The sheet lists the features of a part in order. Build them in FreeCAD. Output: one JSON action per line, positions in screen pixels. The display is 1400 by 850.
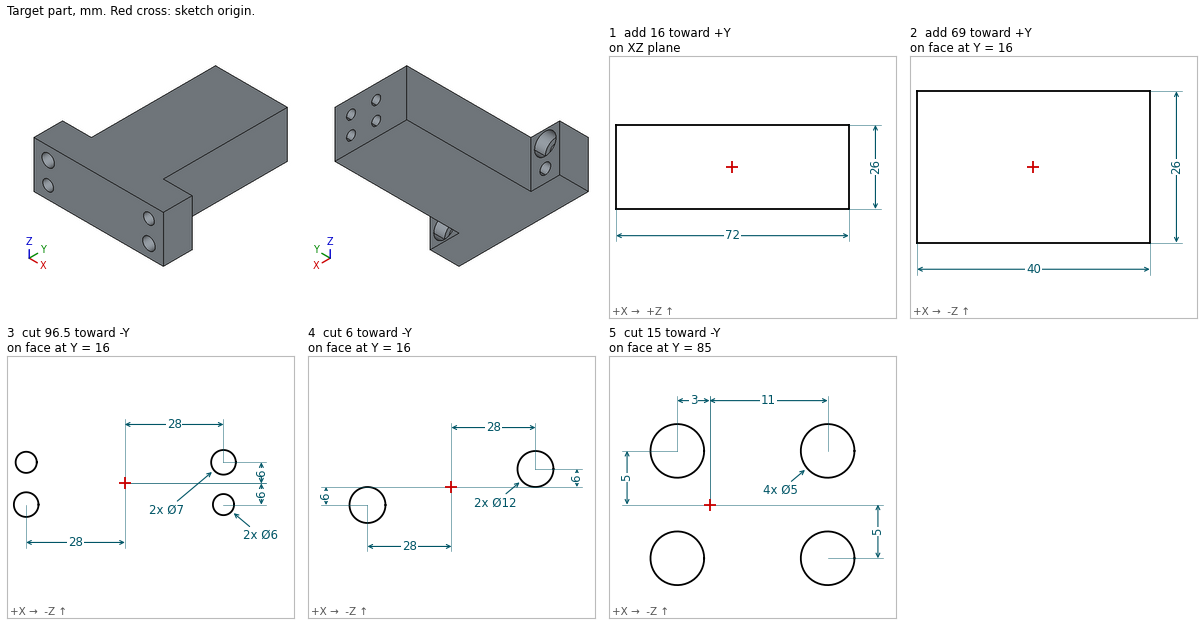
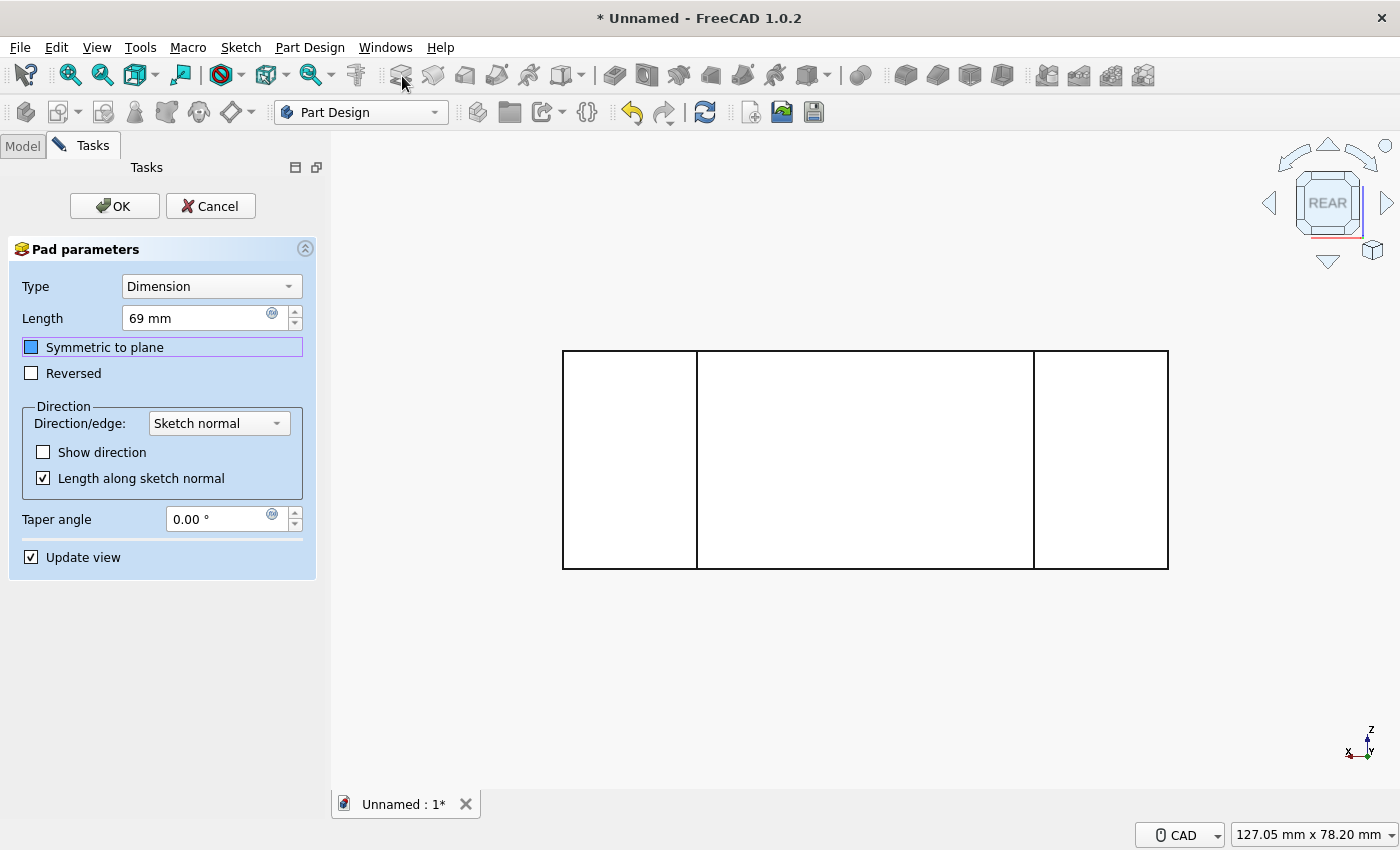
{"action": "left_click", "coordinate": [115, 206]}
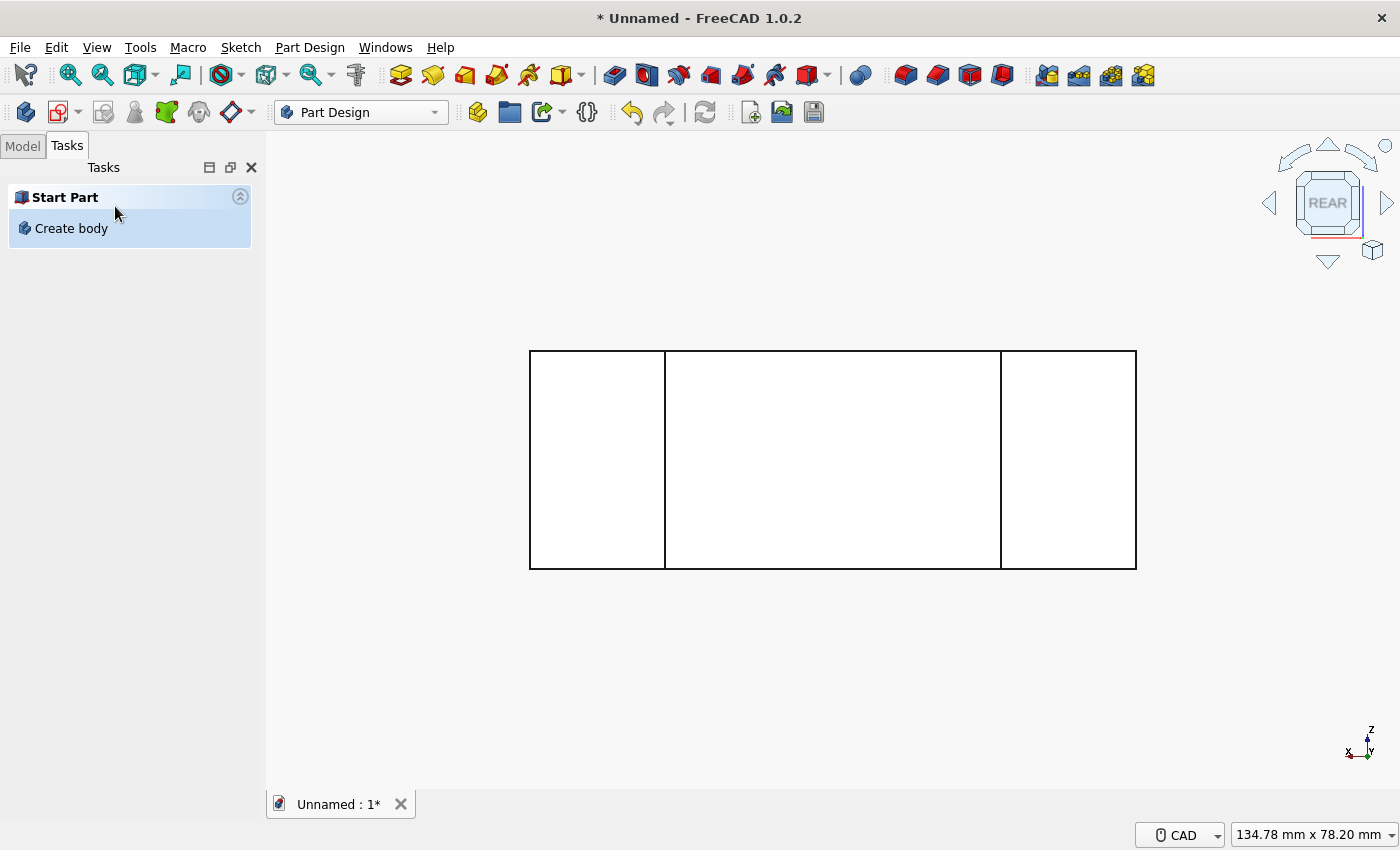
{"action": "left_click", "coordinate": [597, 428]}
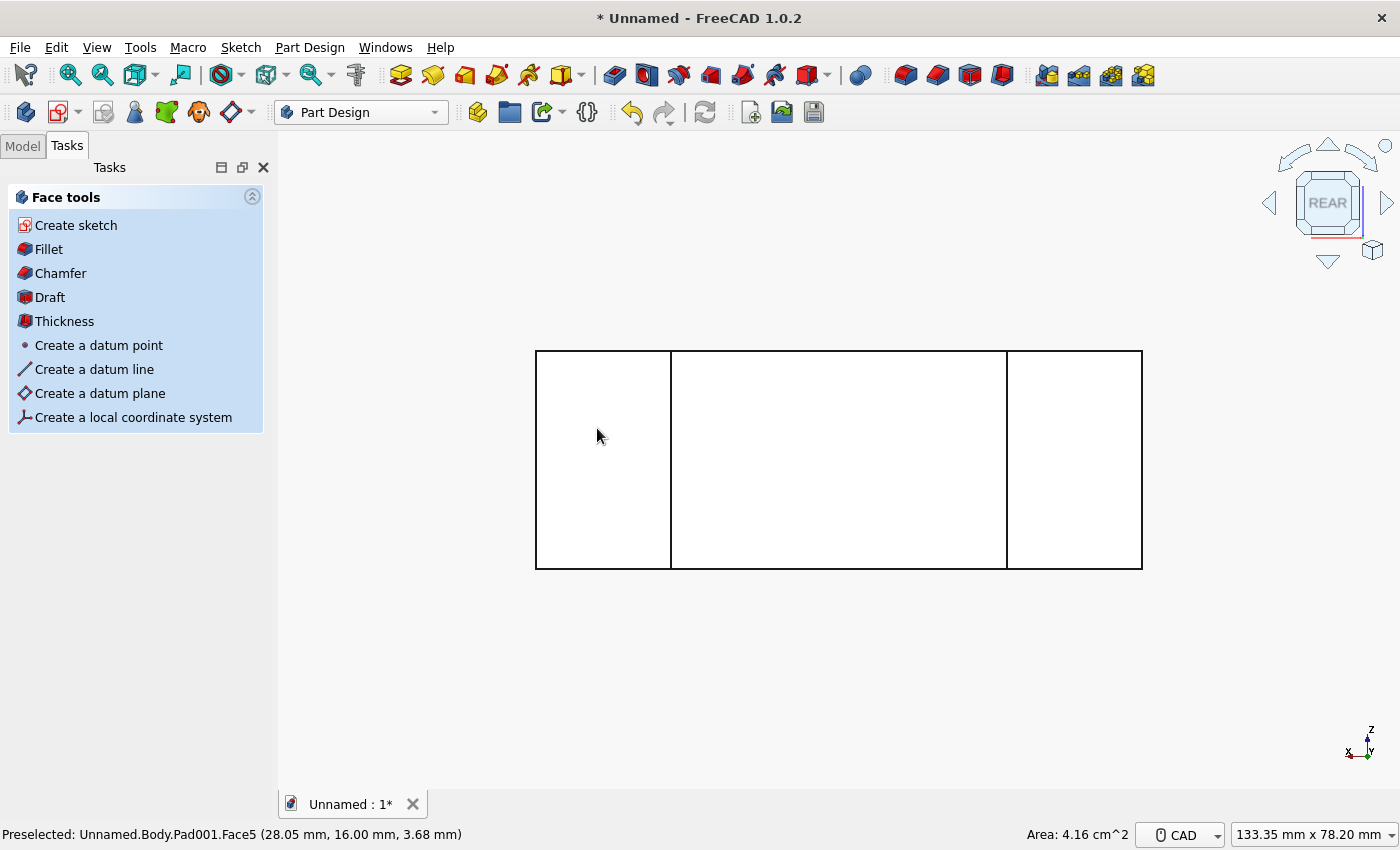
{"action": "left_click", "coordinate": [58, 112]}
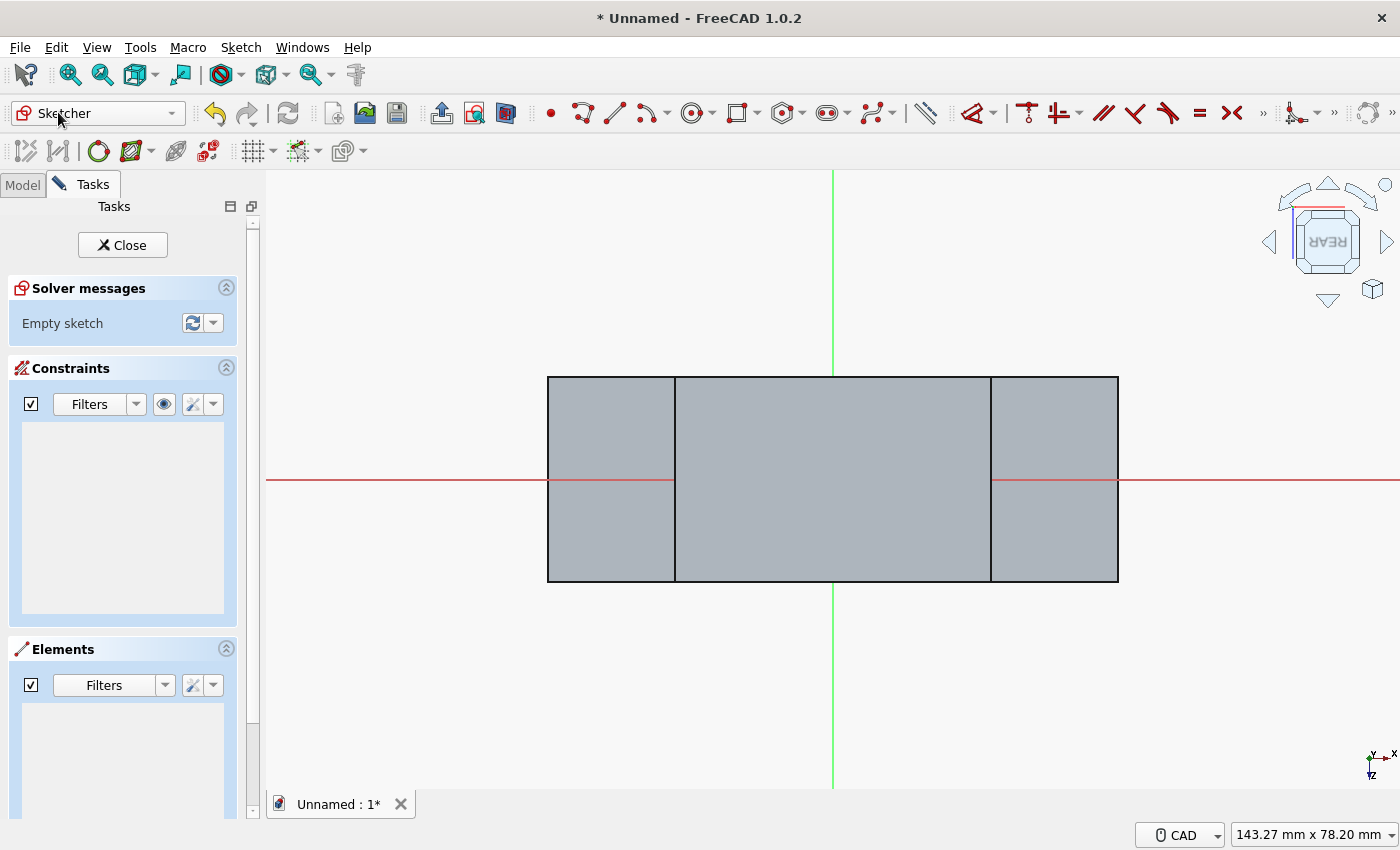
{"action": "key", "text": "g c"}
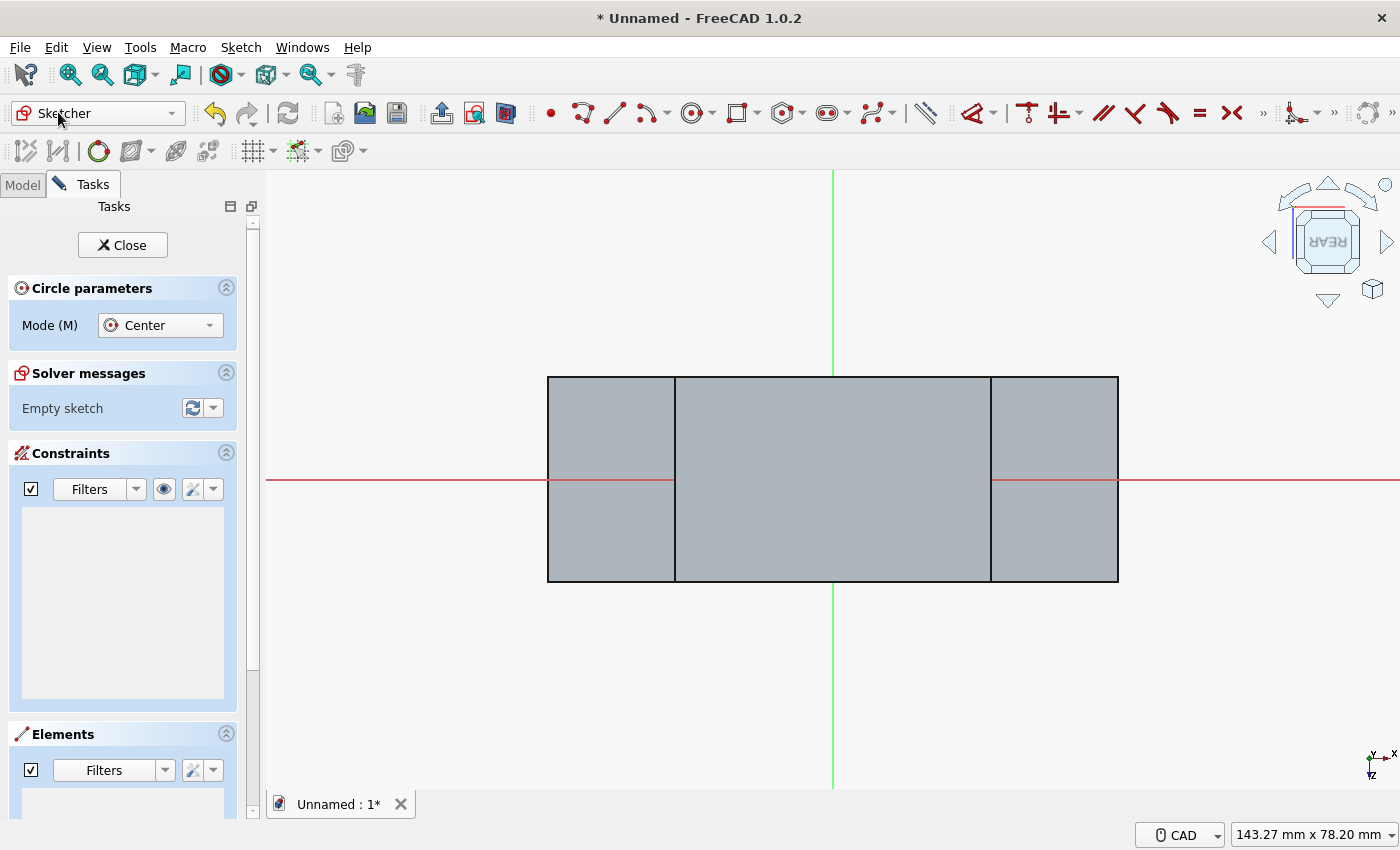
{"action": "left_click", "coordinate": [1055, 432]}
{"action": "mouse_move", "coordinate": [1074, 412]}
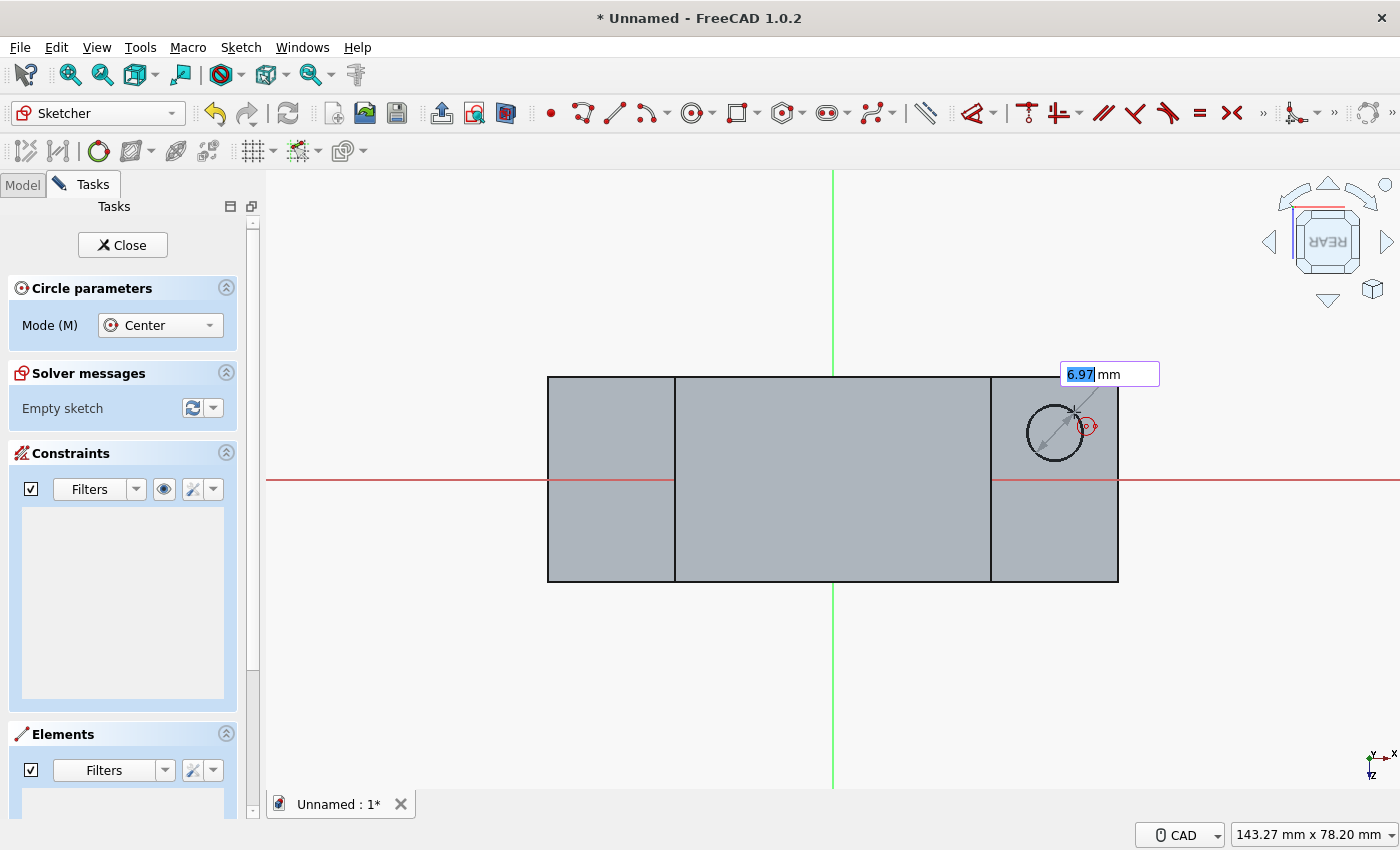
{"action": "type", "text": "7"}
{"action": "key", "text": "Return"}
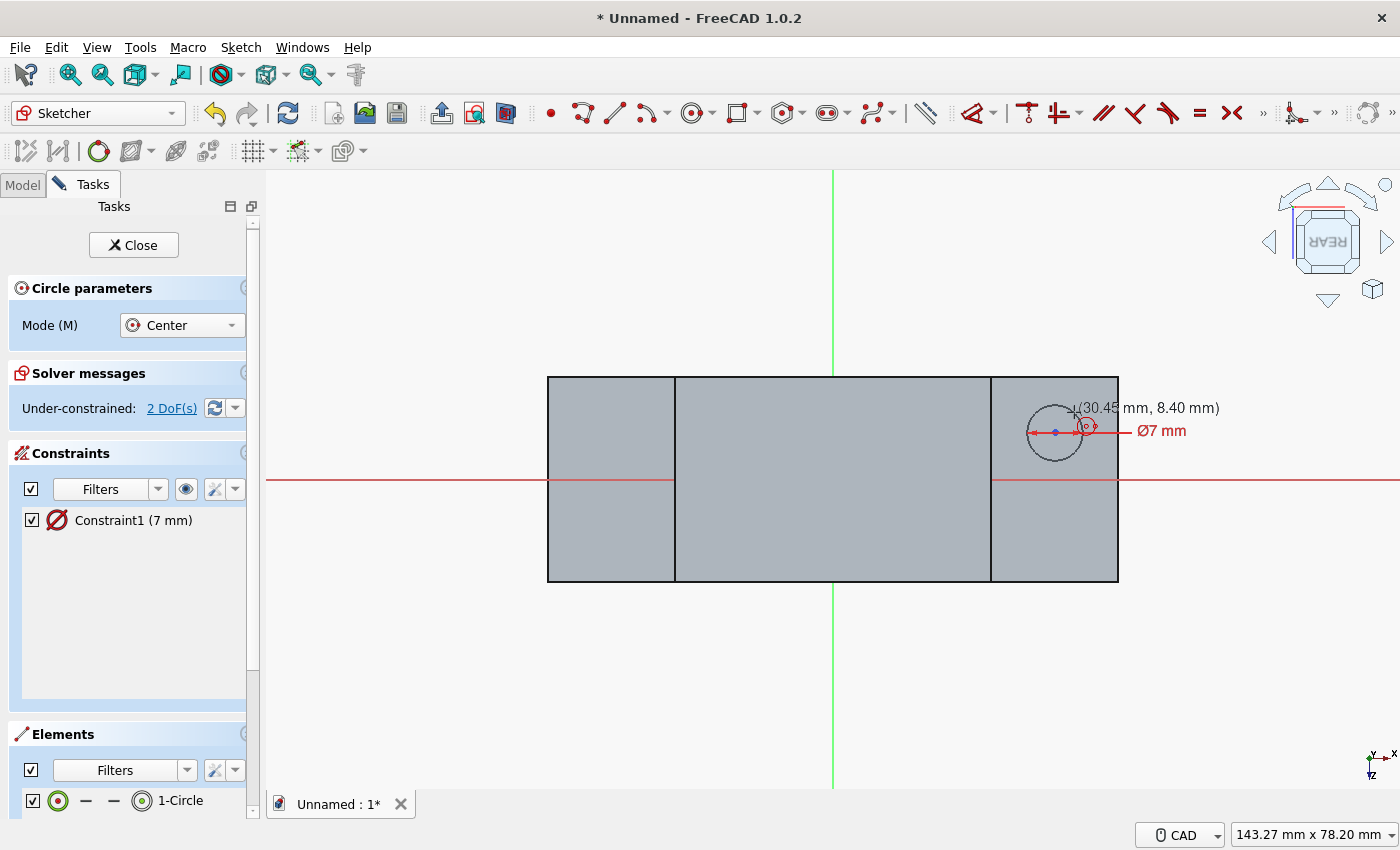
{"action": "left_click", "coordinate": [1055, 527]}
{"action": "mouse_move", "coordinate": [1071, 510]}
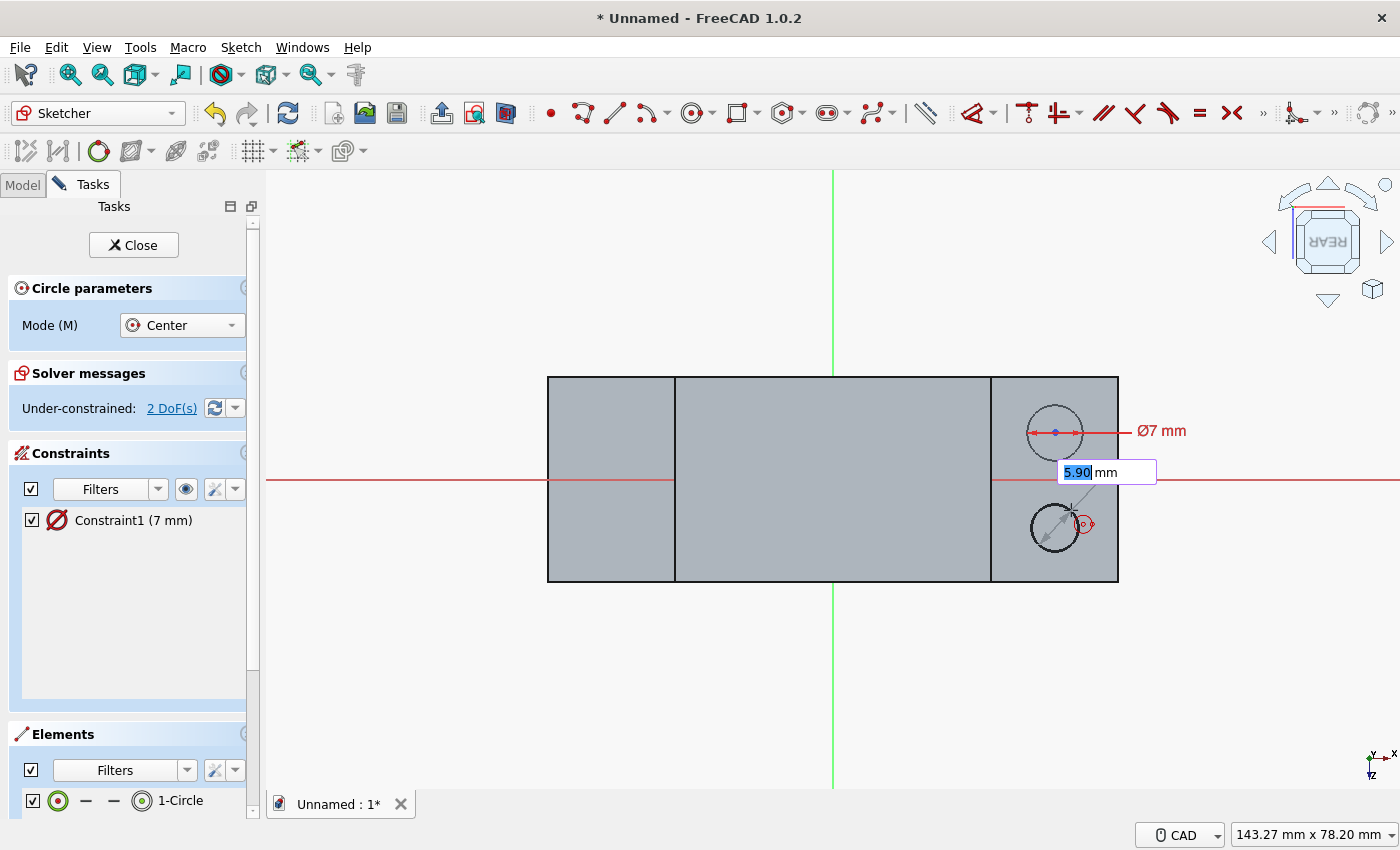
{"action": "type", "text": "6"}
{"action": "key", "text": "Return"}